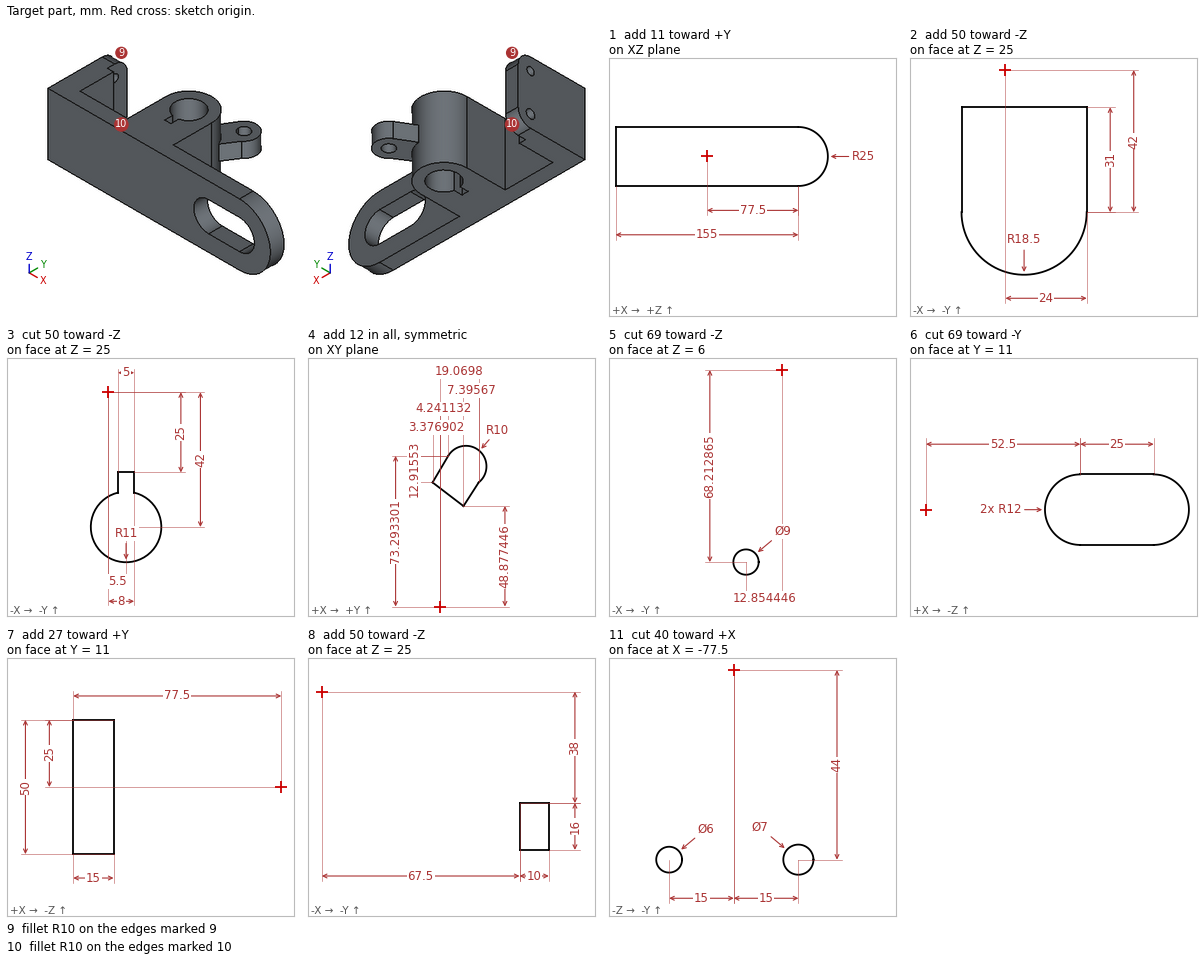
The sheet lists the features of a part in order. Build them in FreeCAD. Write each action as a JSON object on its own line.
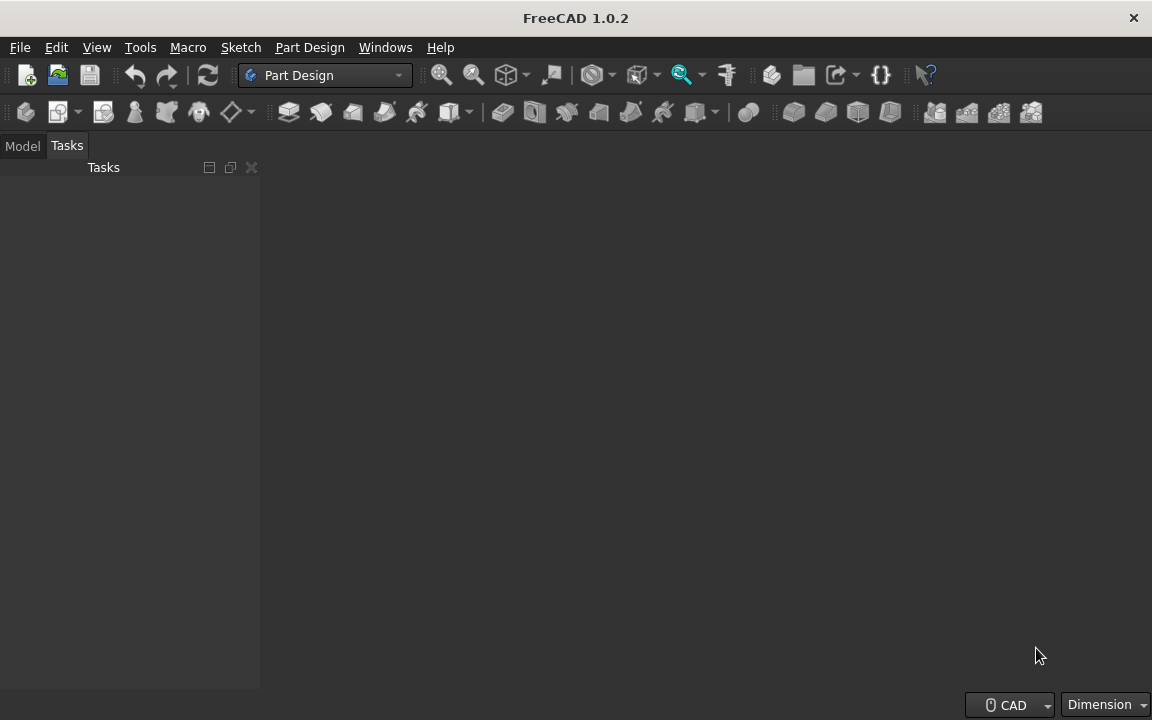
{"action": "left_click", "coordinate": [26, 76]}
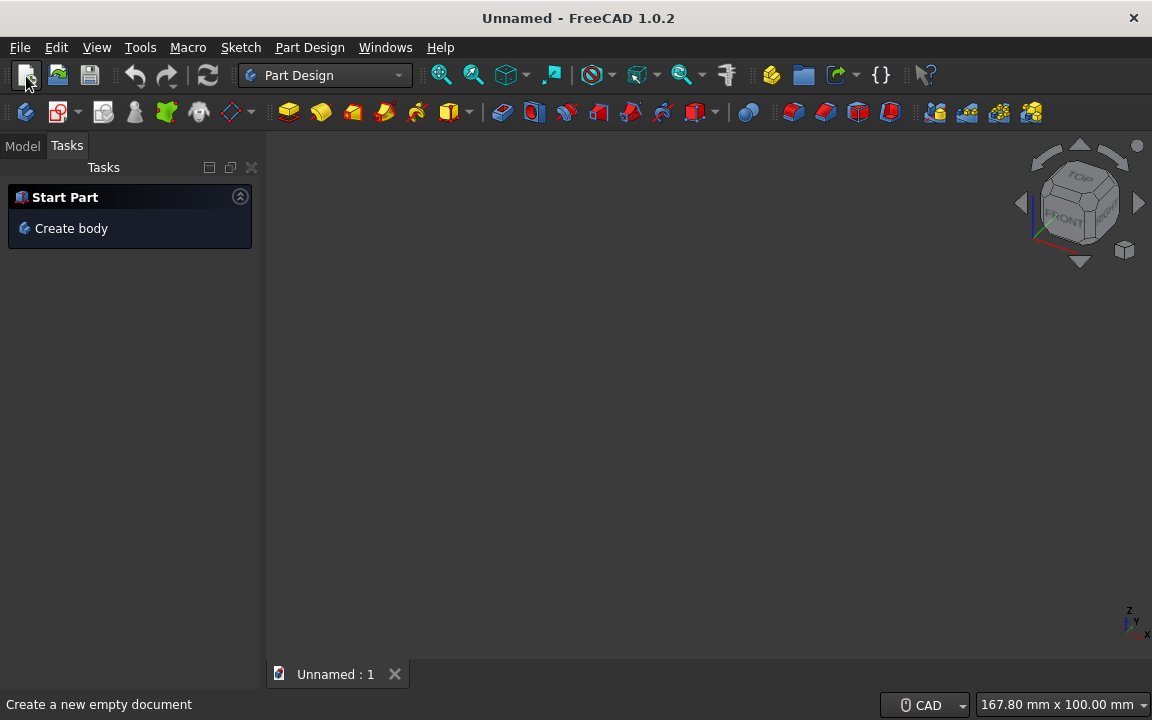
{"action": "left_click", "coordinate": [58, 112]}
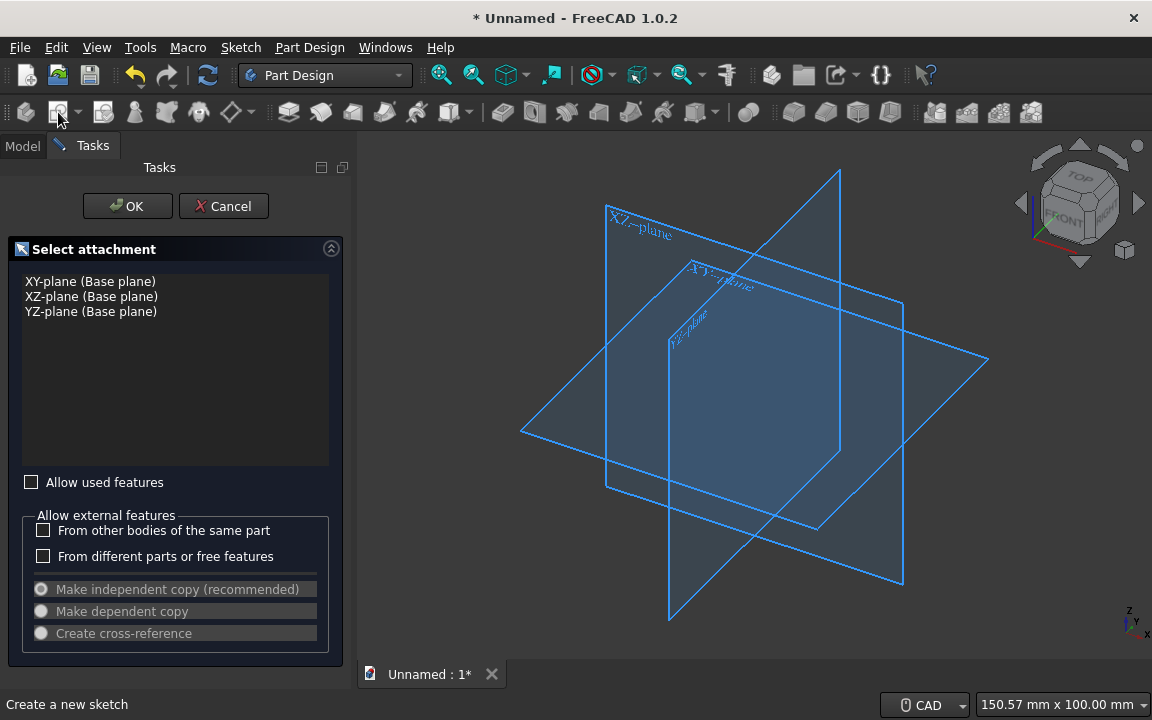
{"action": "left_click", "coordinate": [82, 296]}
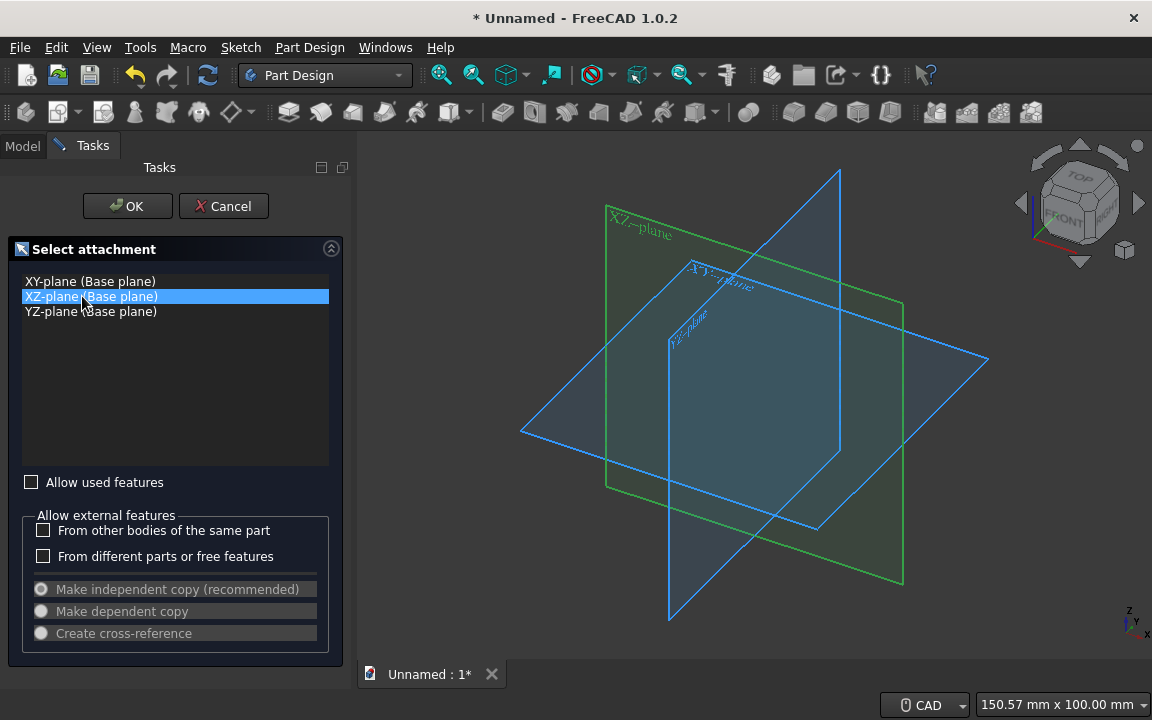
{"action": "left_click", "coordinate": [128, 206]}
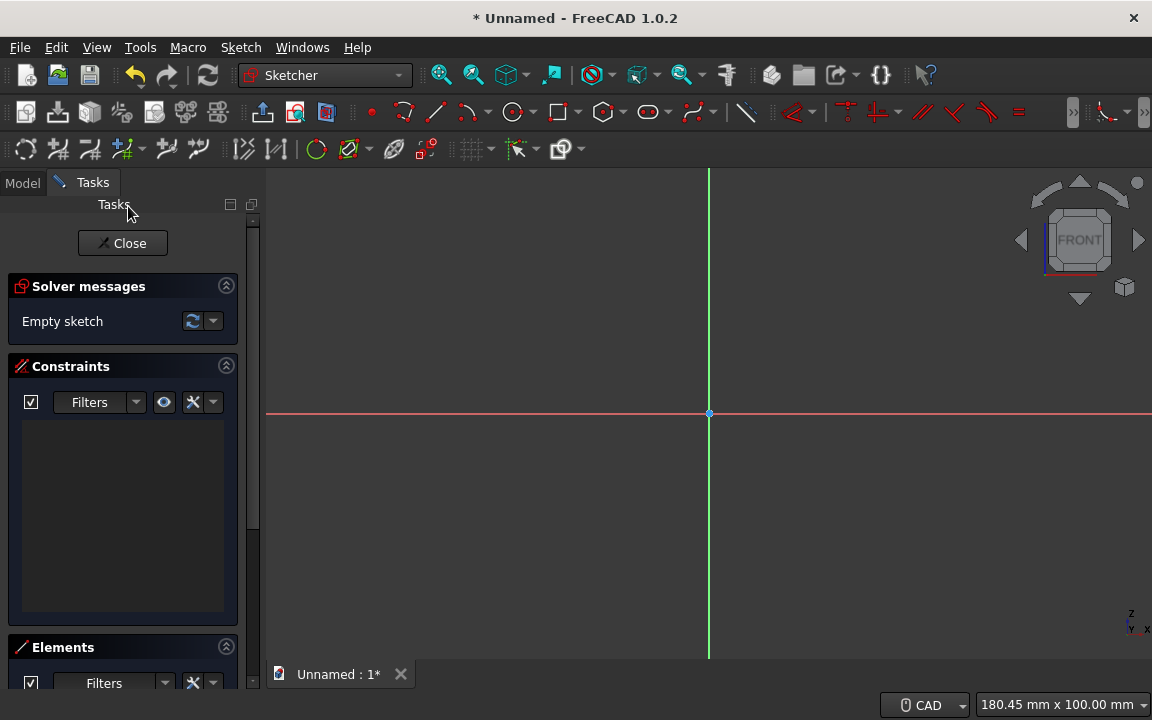
{"action": "scroll", "coordinate": [483, 414], "scroll_direction": "down", "scroll_amount": 3}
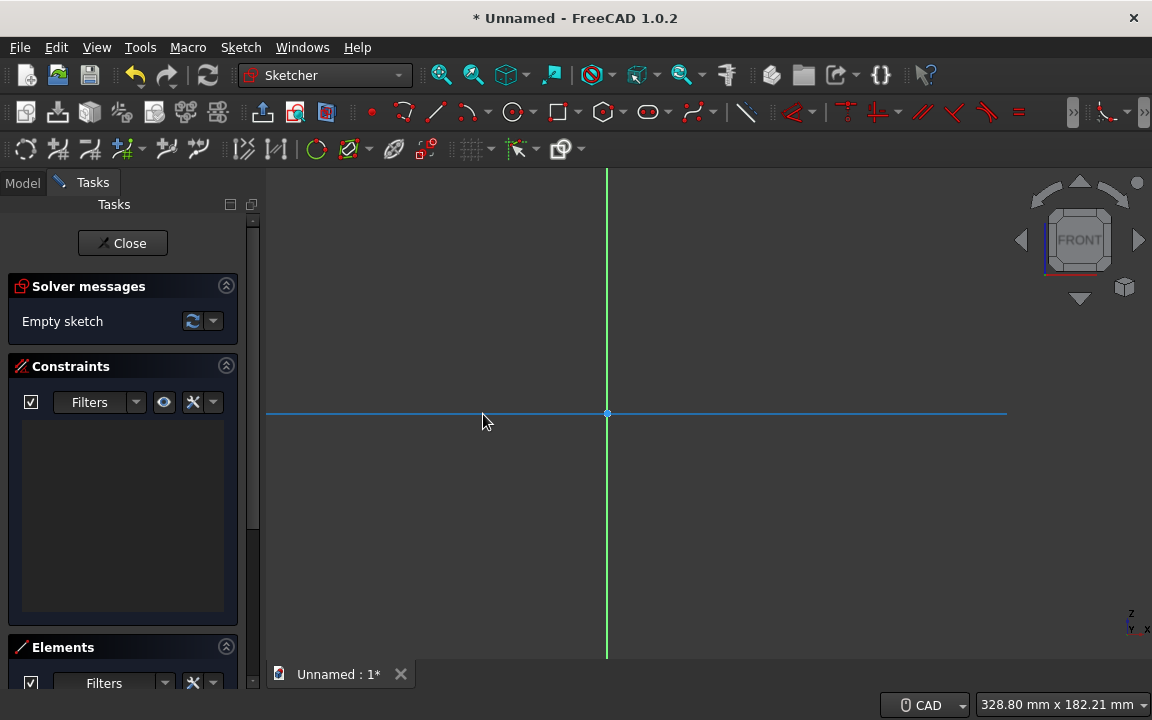
{"action": "left_click", "coordinate": [404, 112]}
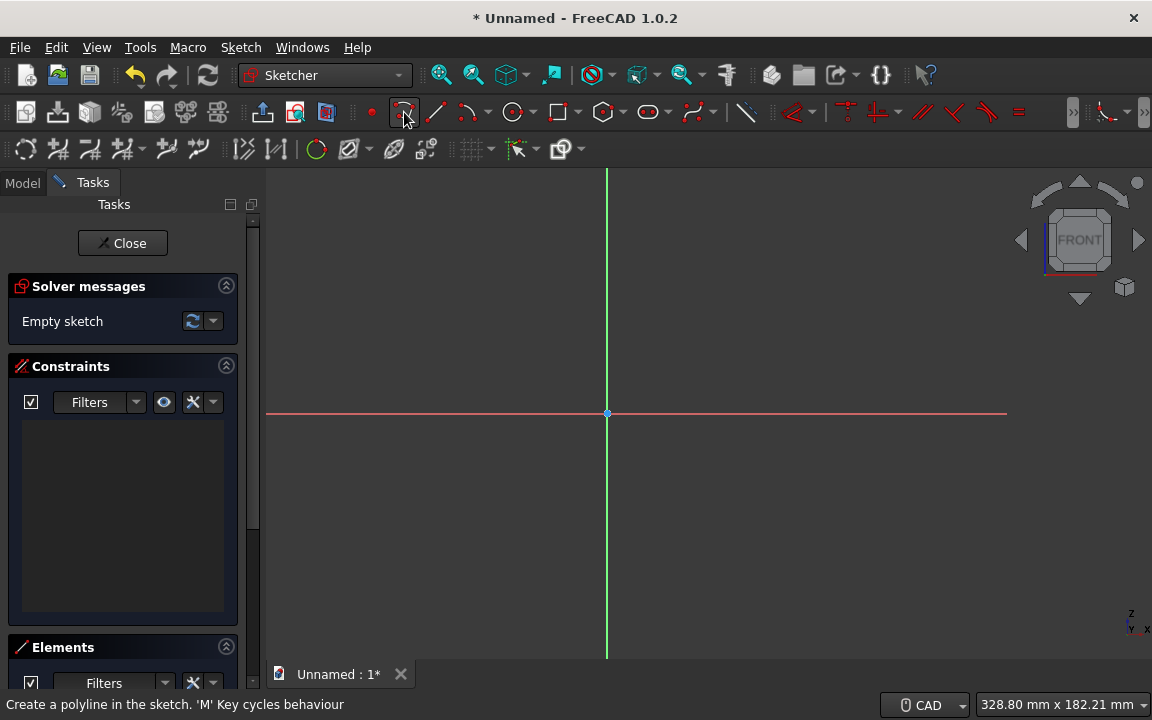
{"action": "left_click", "coordinate": [816, 481]}
{"action": "left_click", "coordinate": [398, 481]}
{"action": "left_click", "coordinate": [398, 347]}
{"action": "left_click", "coordinate": [816, 347]}
{"action": "right_click", "coordinate": [816, 347]}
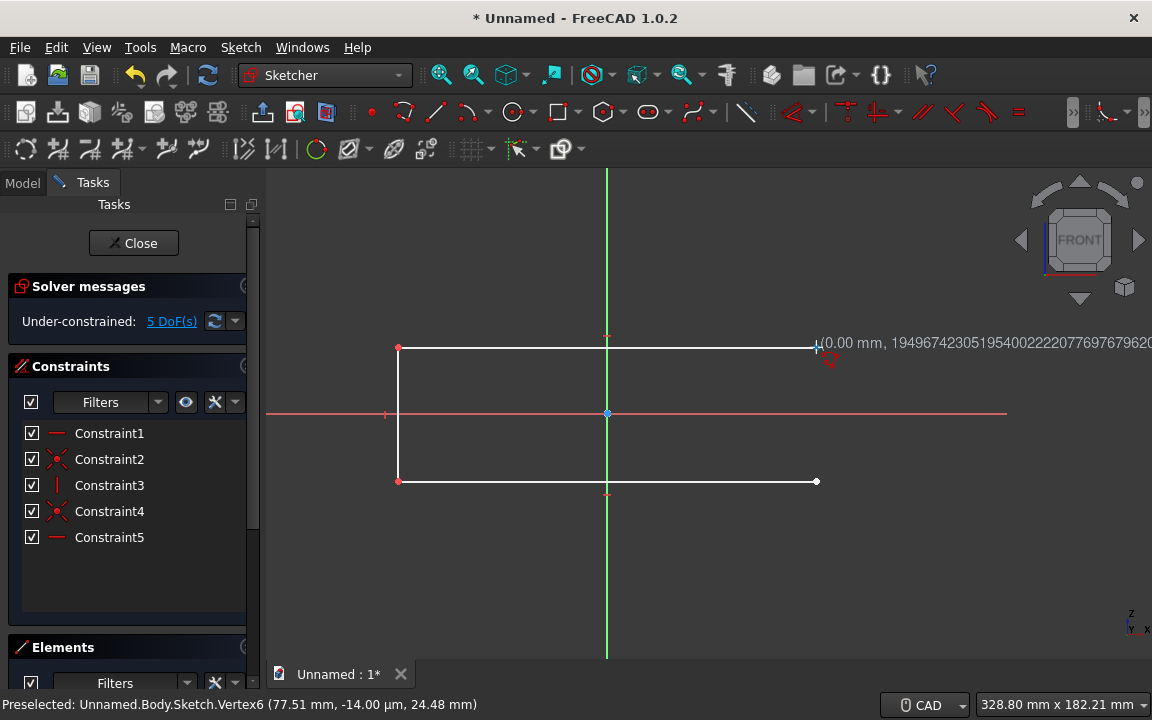
{"action": "key", "text": "g 3 a"}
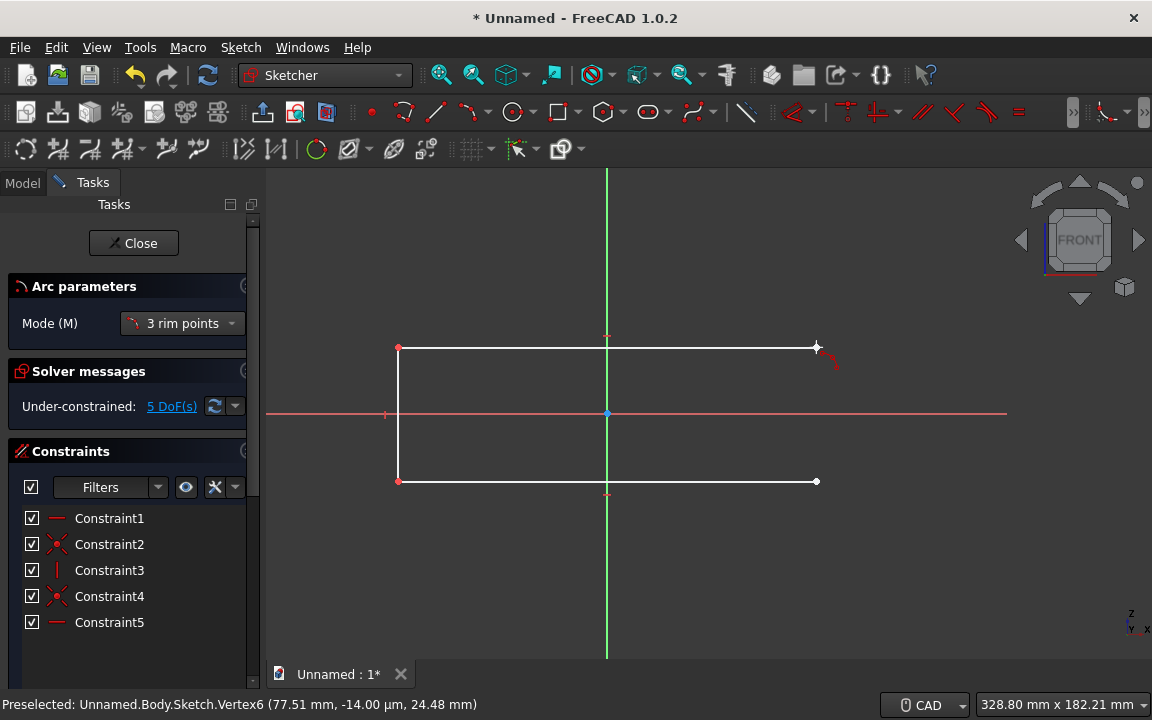
{"action": "left_click", "coordinate": [816, 348]}
{"action": "left_click", "coordinate": [816, 482]}
{"action": "left_click", "coordinate": [880, 435]}
{"action": "key", "text": "Escape"}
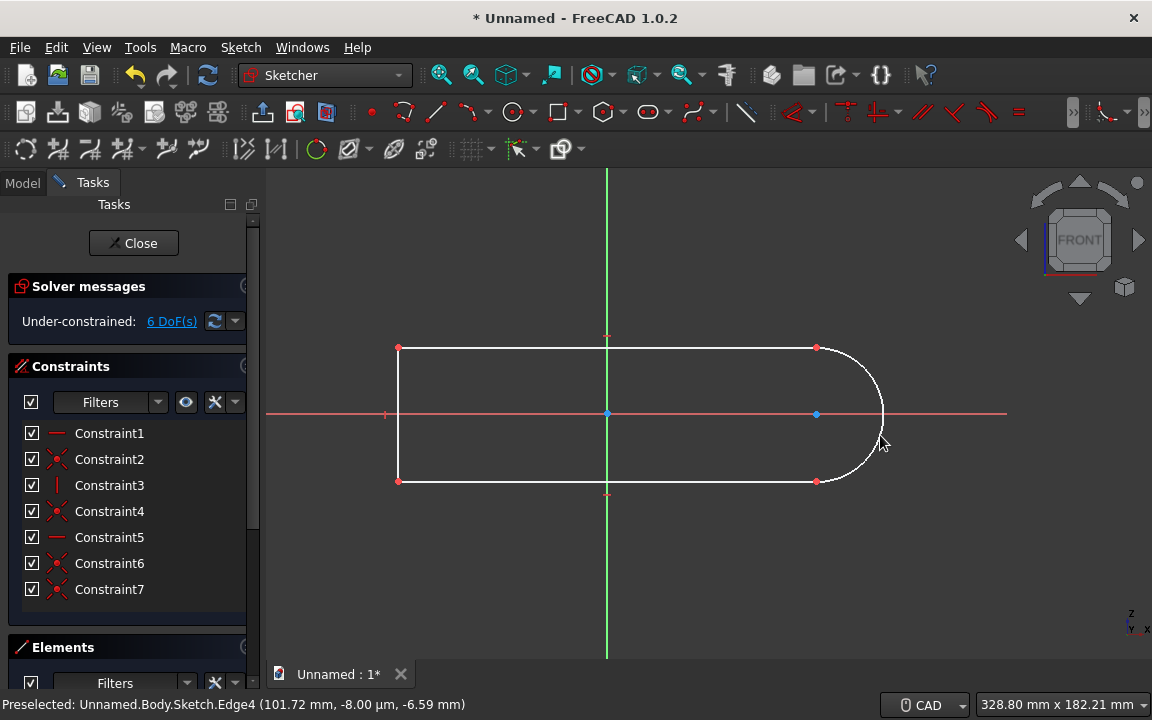
{"action": "left_click", "coordinate": [691, 482]}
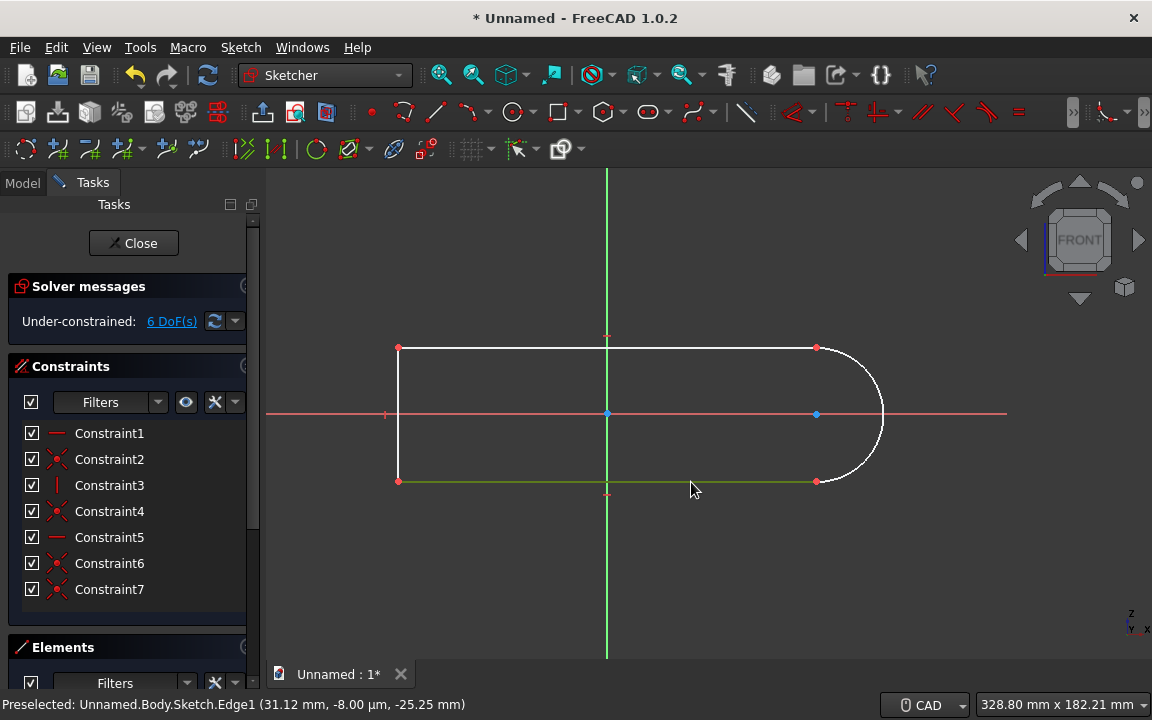
{"action": "left_click", "coordinate": [870, 455]}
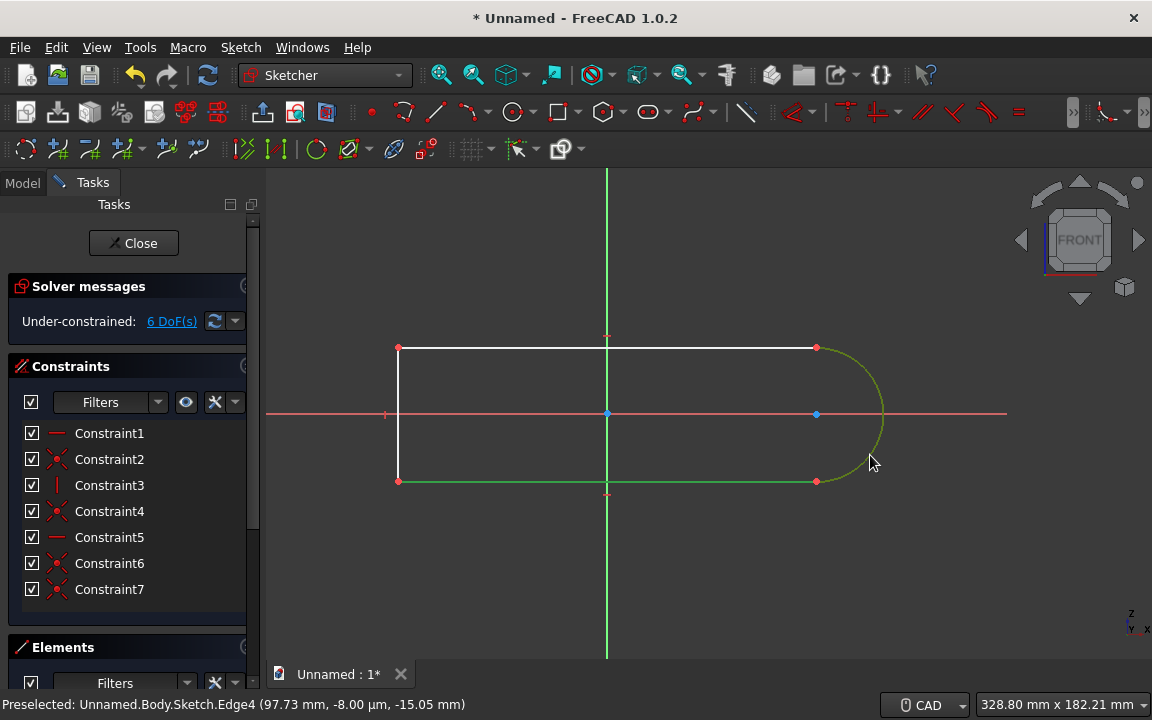
{"action": "left_click", "coordinate": [988, 112]}